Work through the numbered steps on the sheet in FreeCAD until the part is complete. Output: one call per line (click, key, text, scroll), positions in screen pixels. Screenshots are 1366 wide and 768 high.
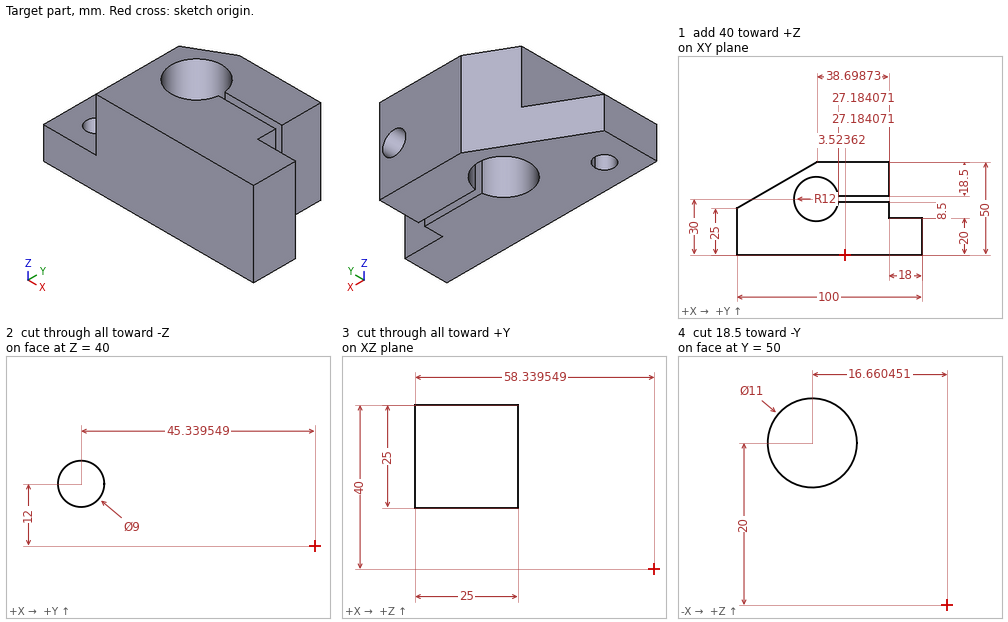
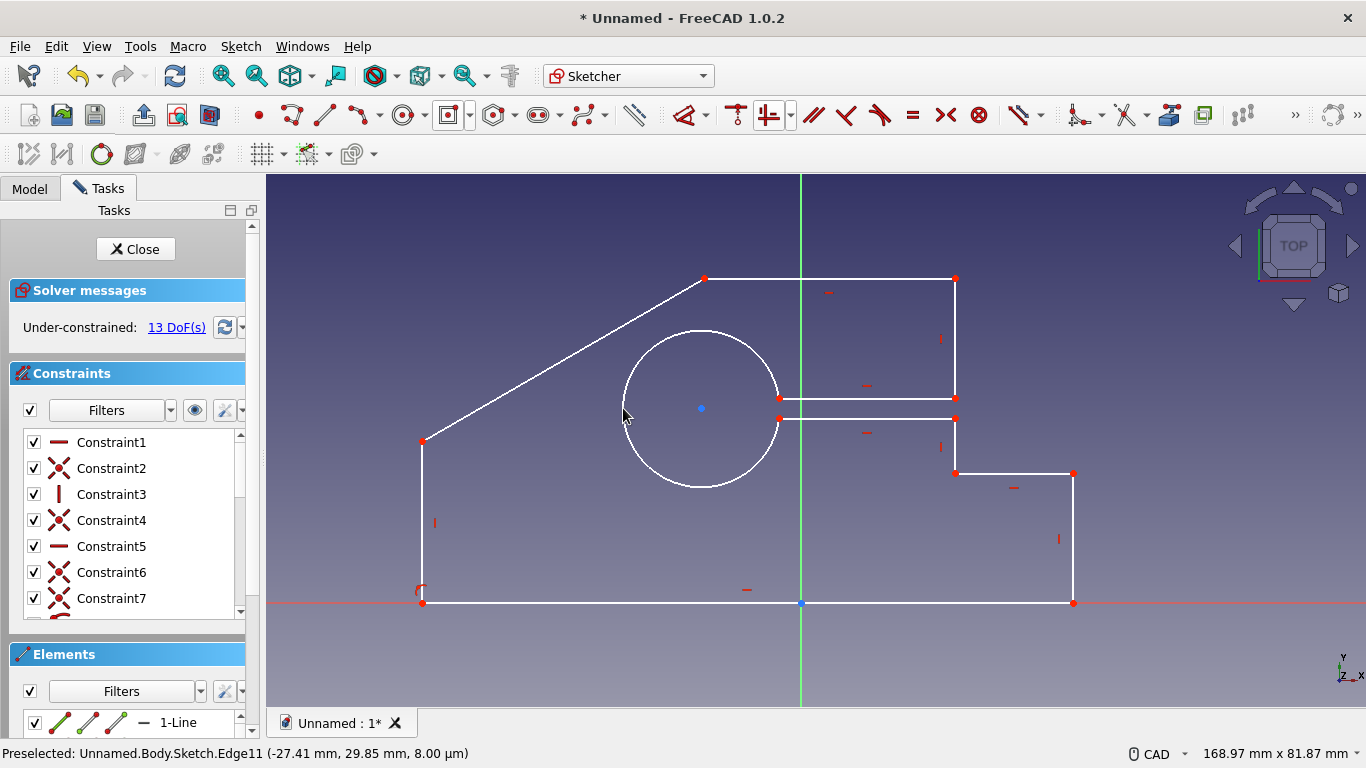
click(684, 116)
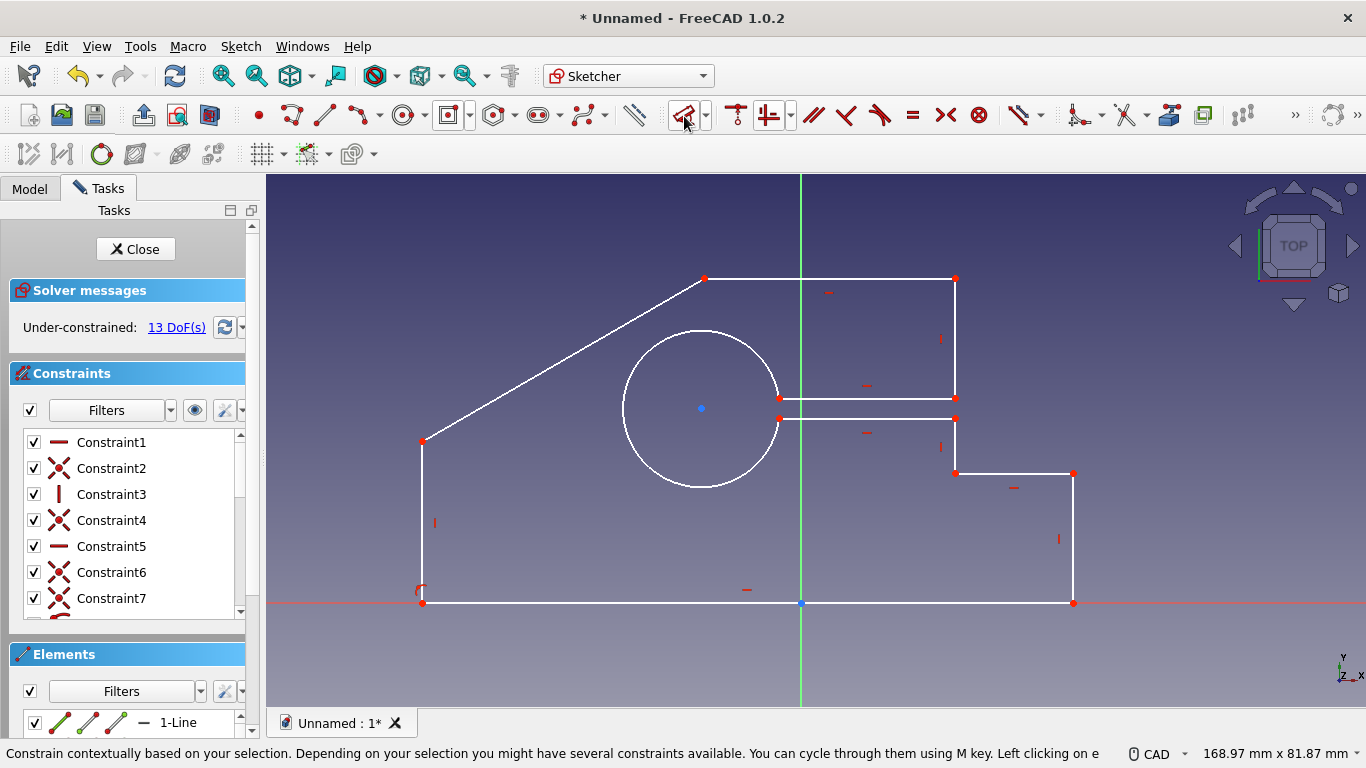
click(673, 336)
click(716, 300)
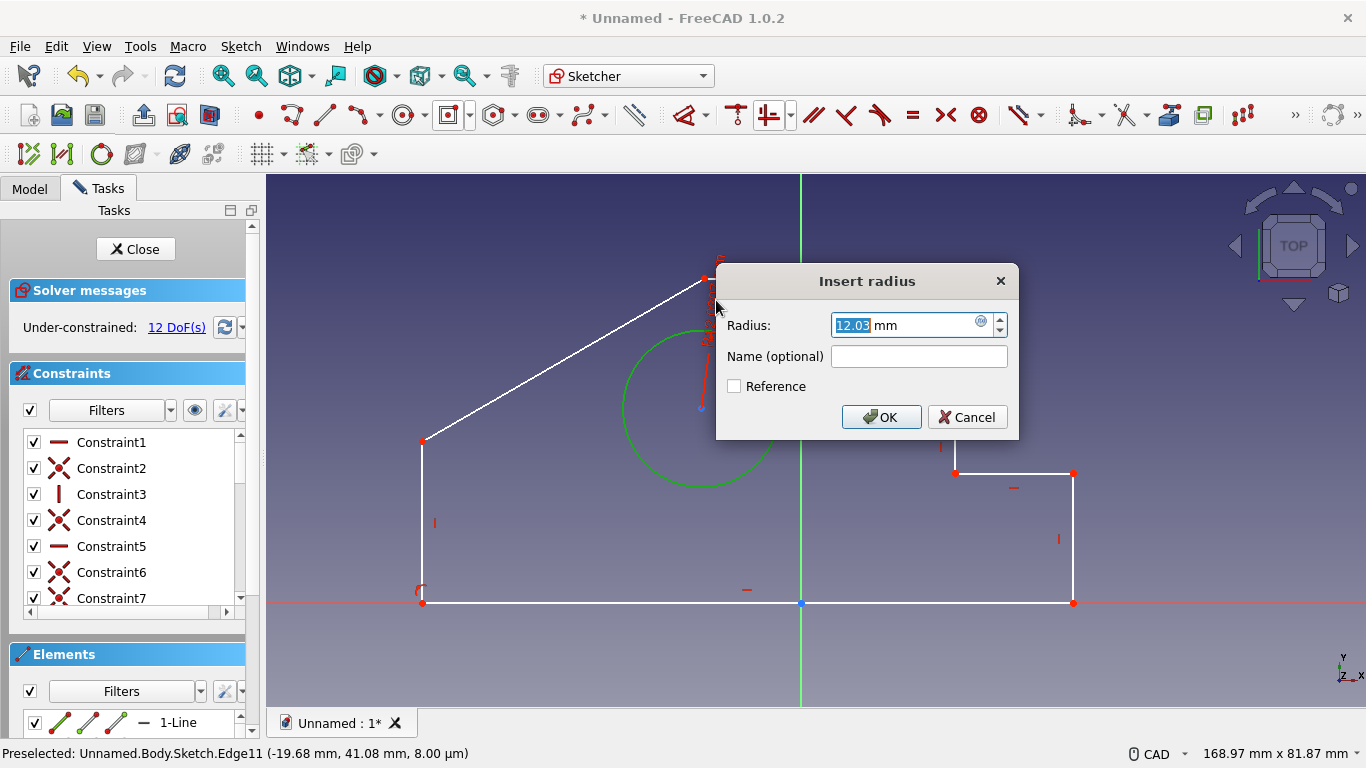
text(12)
key(Return)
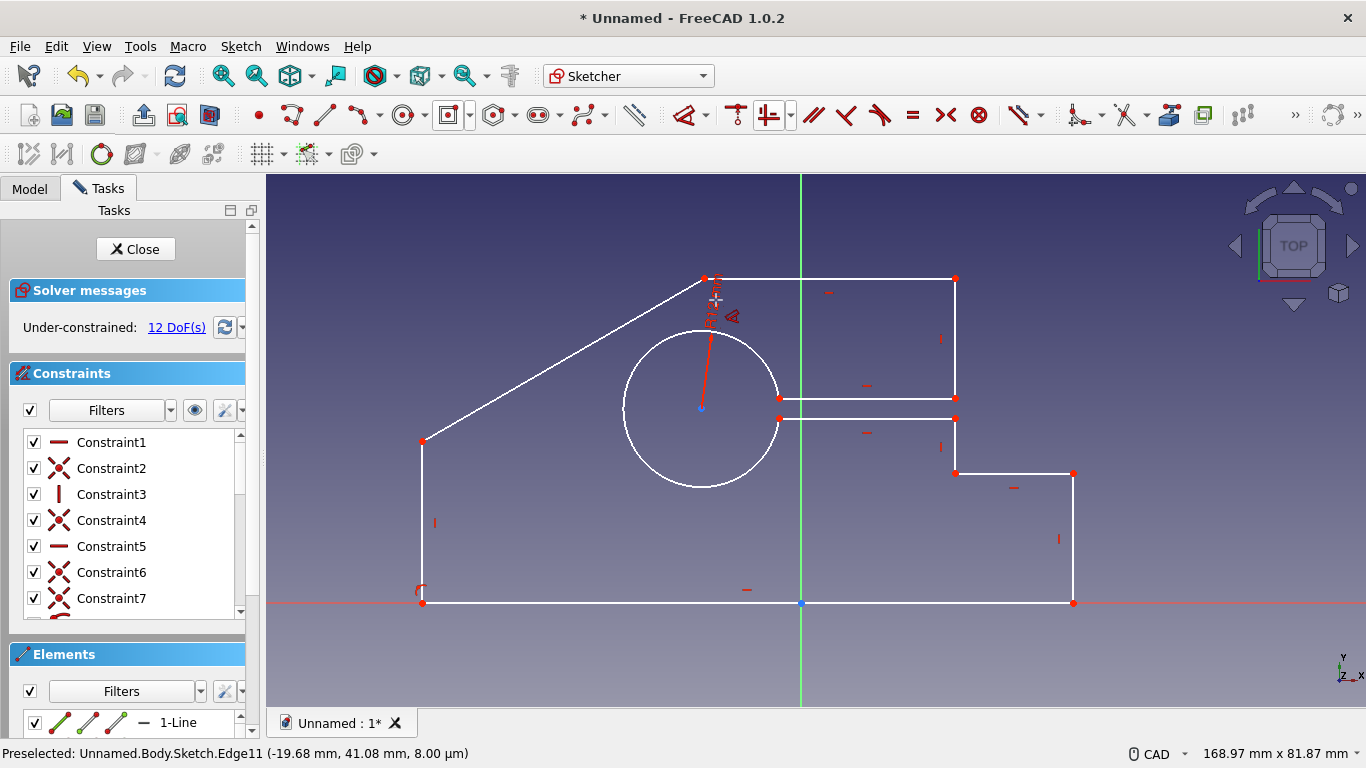
click(422, 490)
click(388, 523)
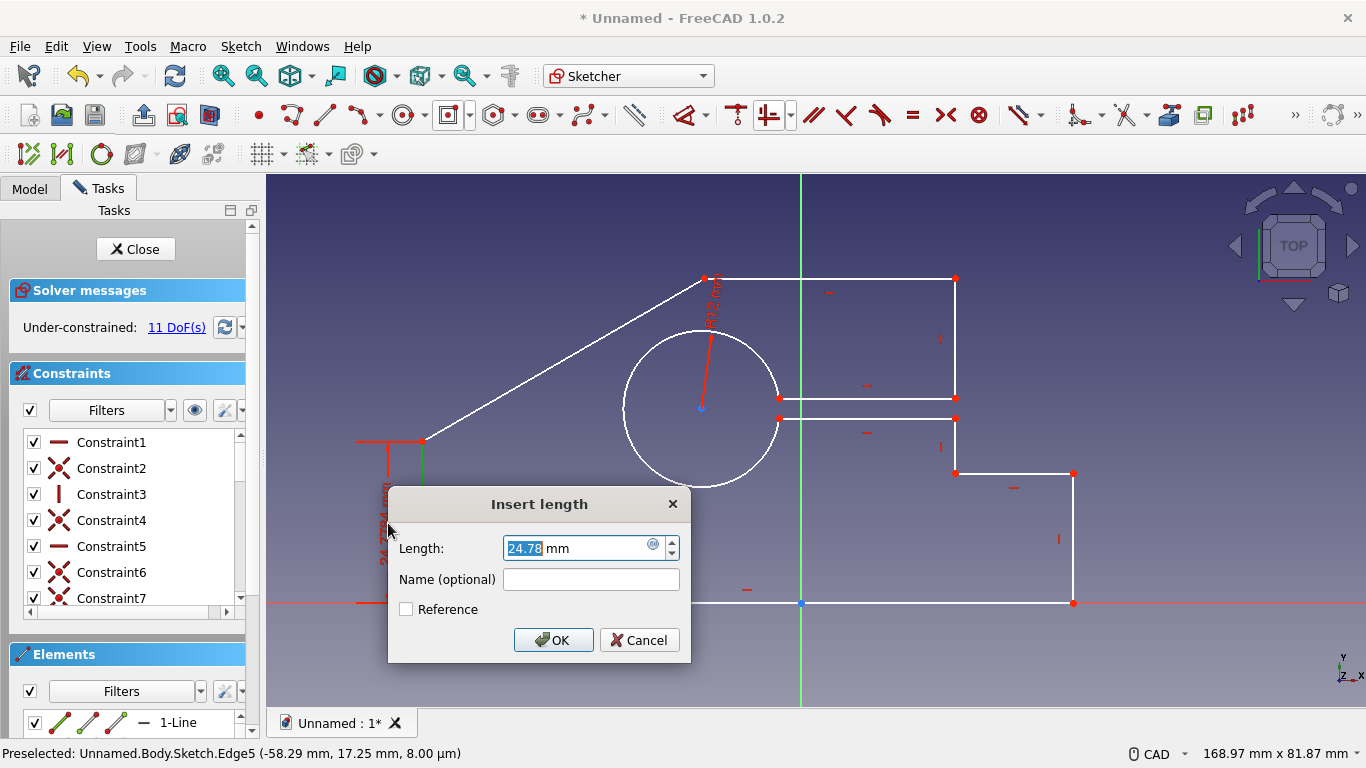
text(25)
key(Return)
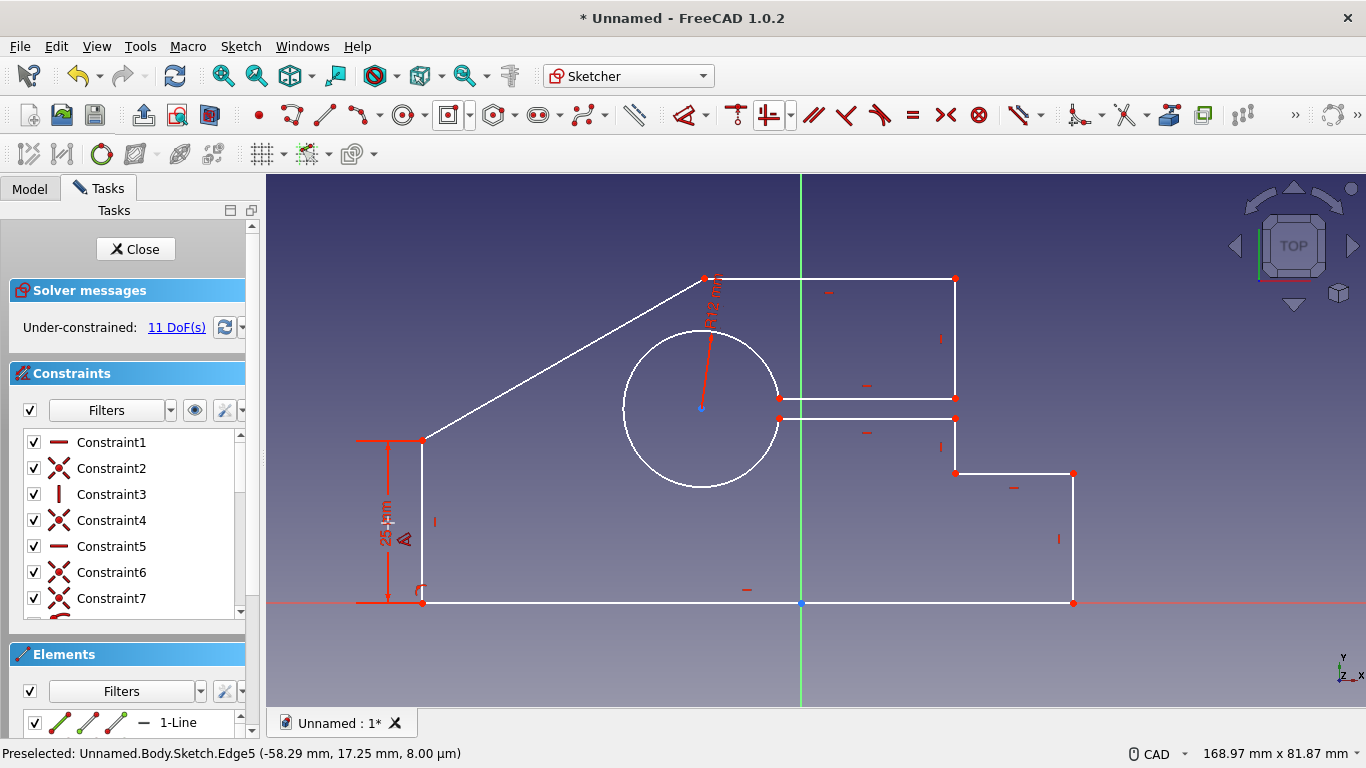
click(1073, 565)
click(1107, 539)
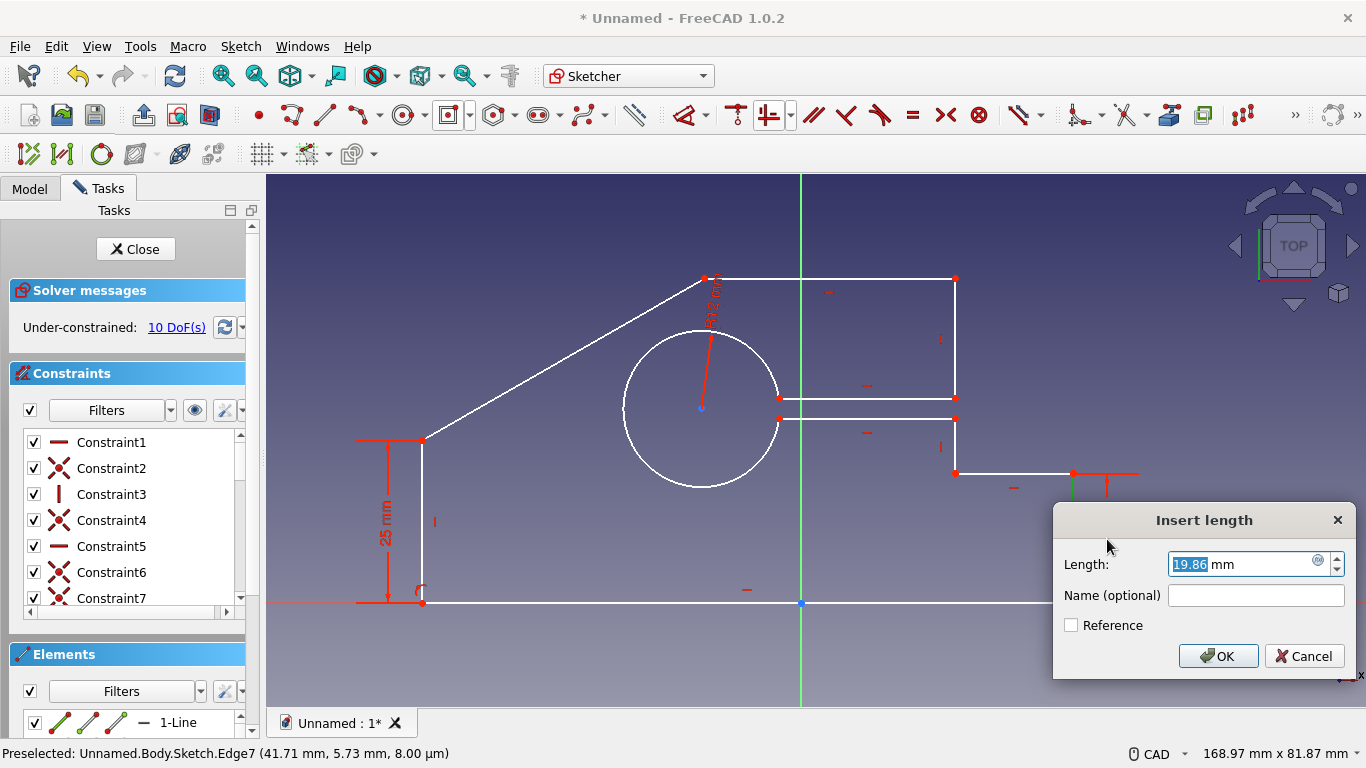
text(20)
key(Return)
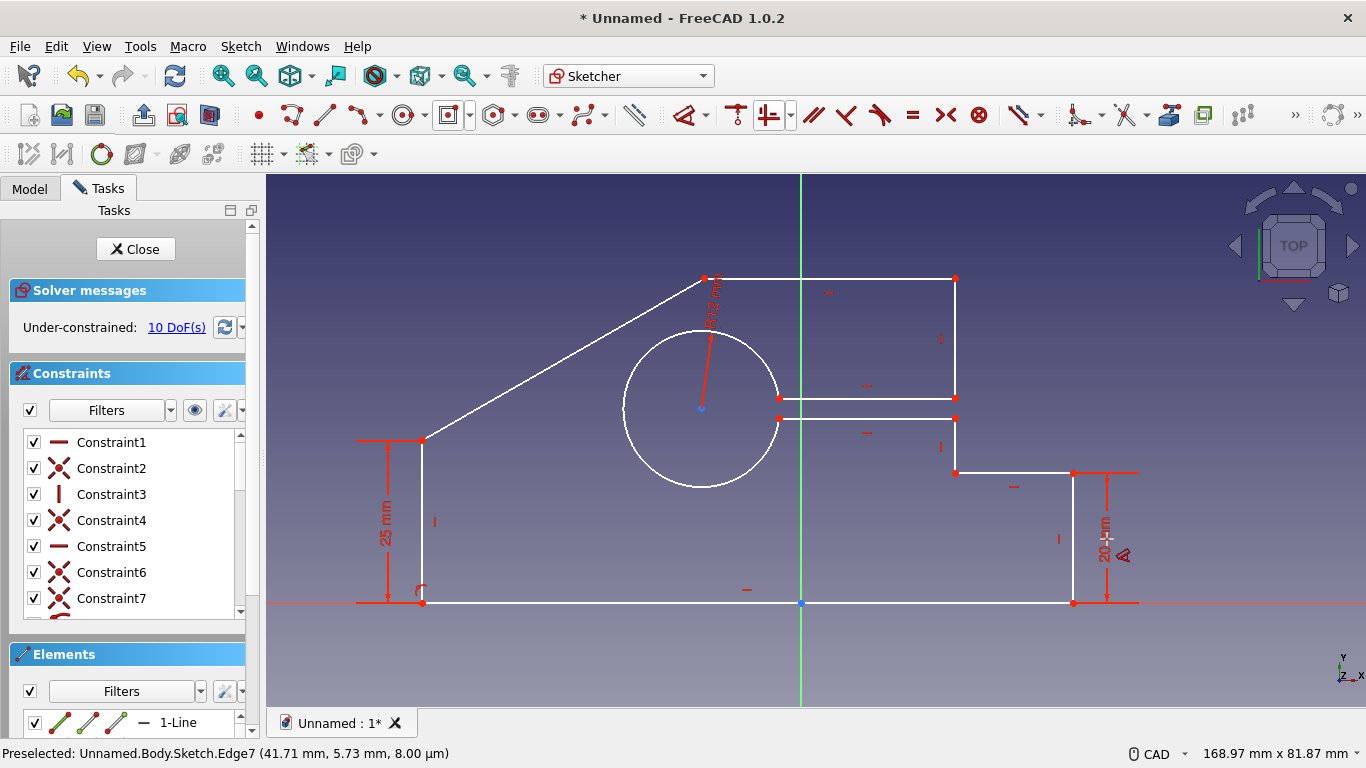
click(1038, 473)
click(1014, 507)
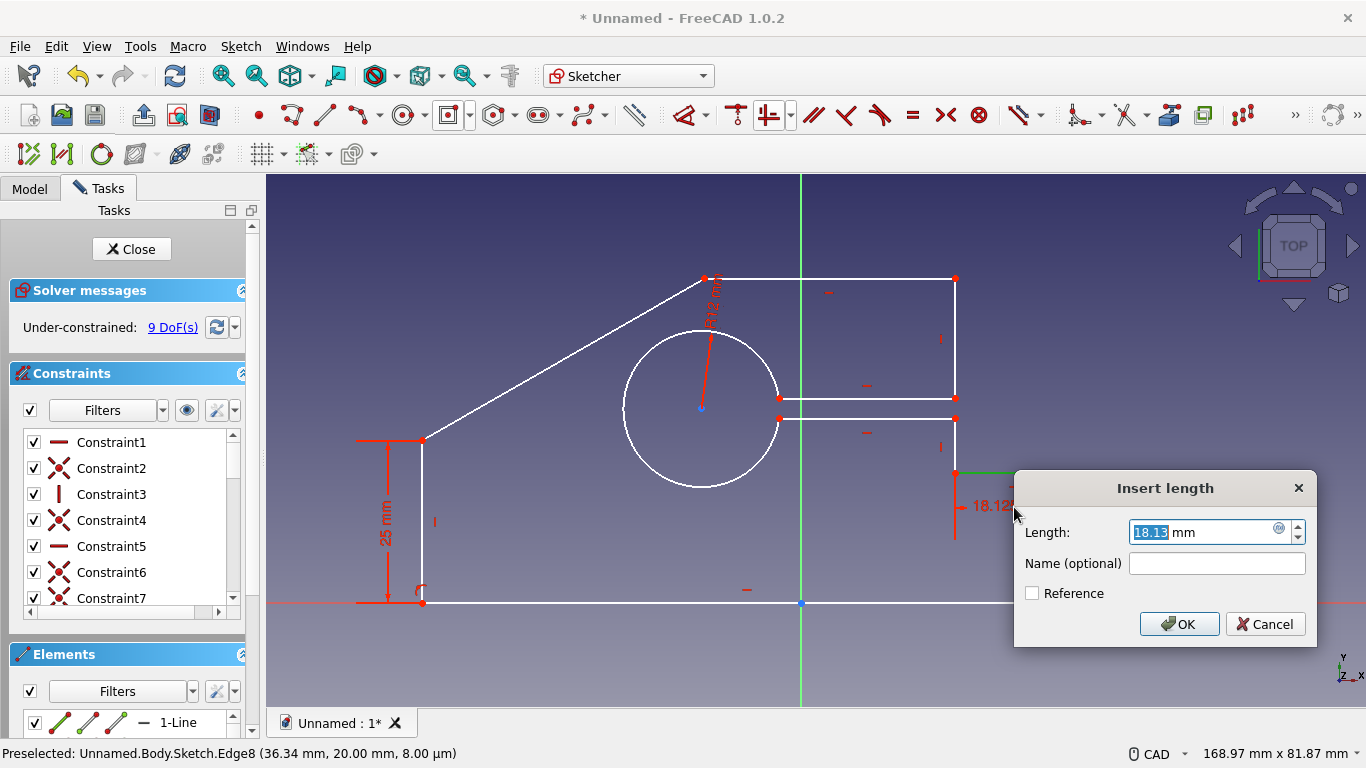
text(18)
key(Return)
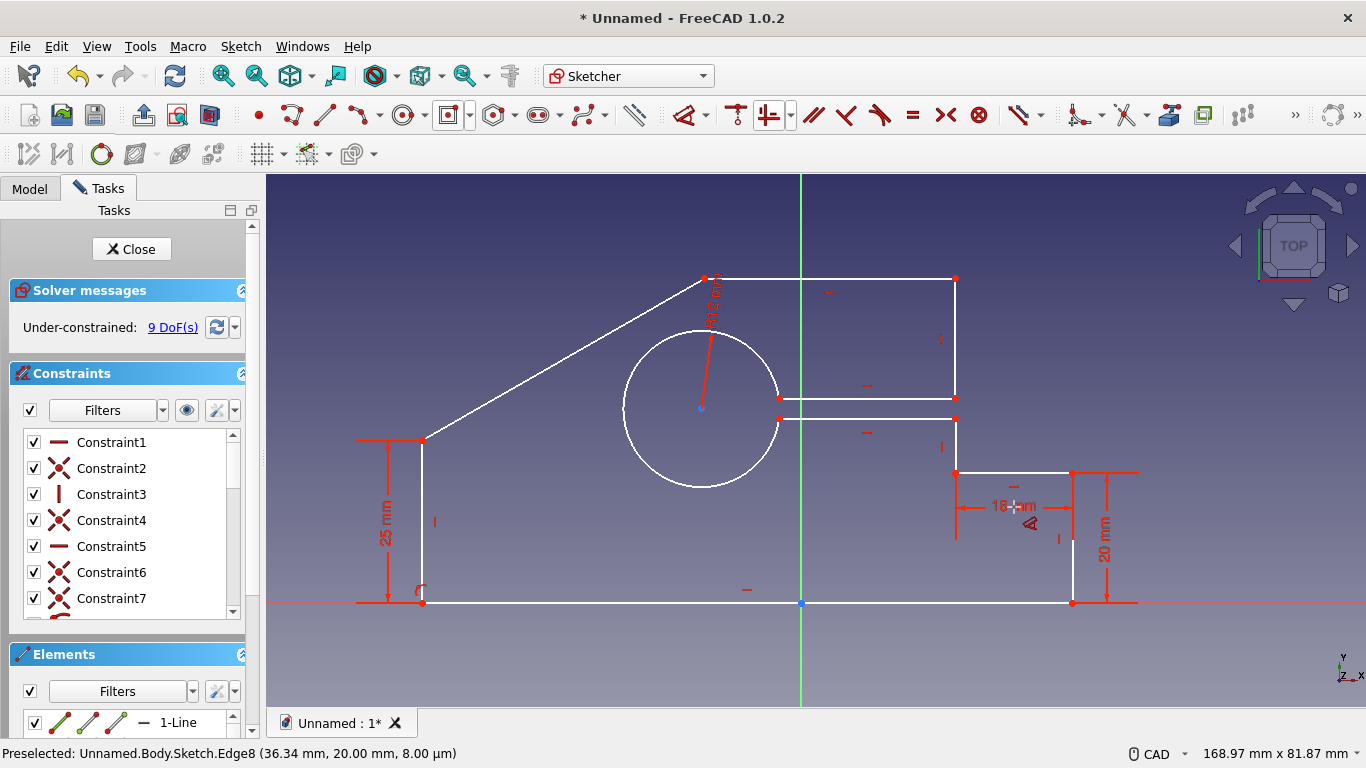
click(617, 603)
click(747, 637)